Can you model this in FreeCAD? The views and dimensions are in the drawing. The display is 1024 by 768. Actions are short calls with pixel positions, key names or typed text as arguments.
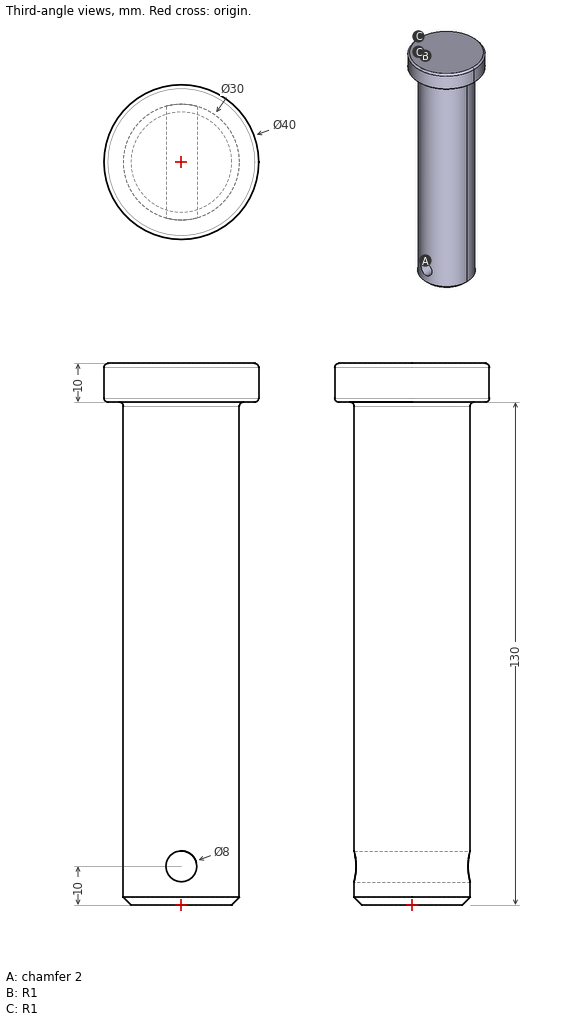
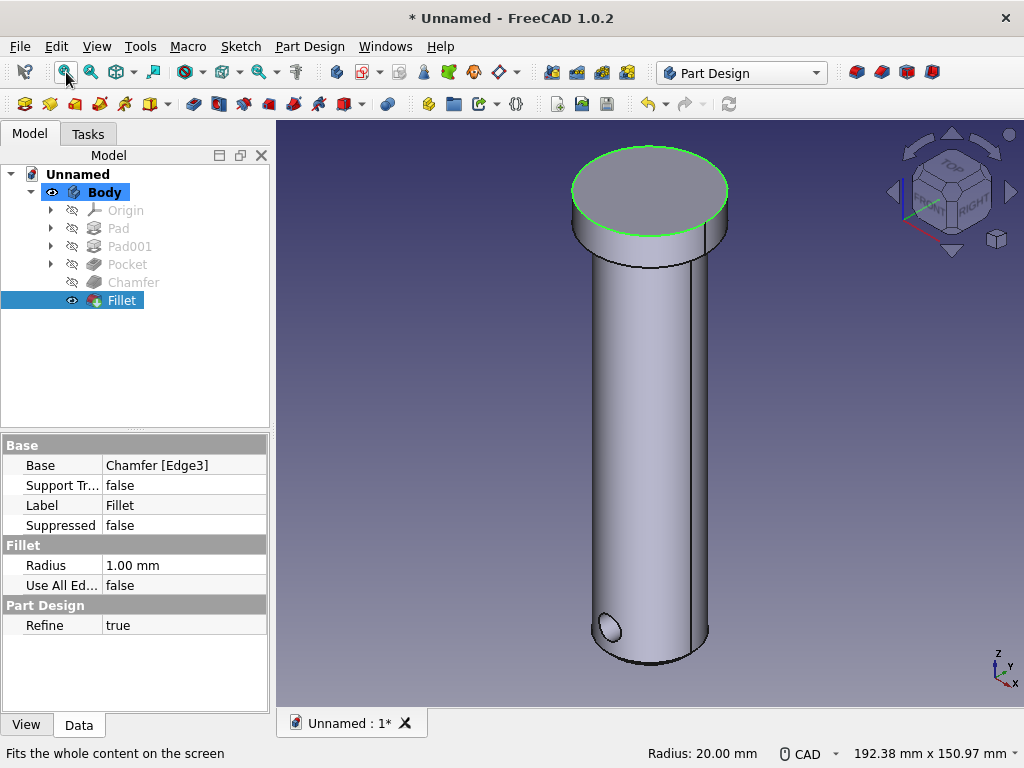
key(1)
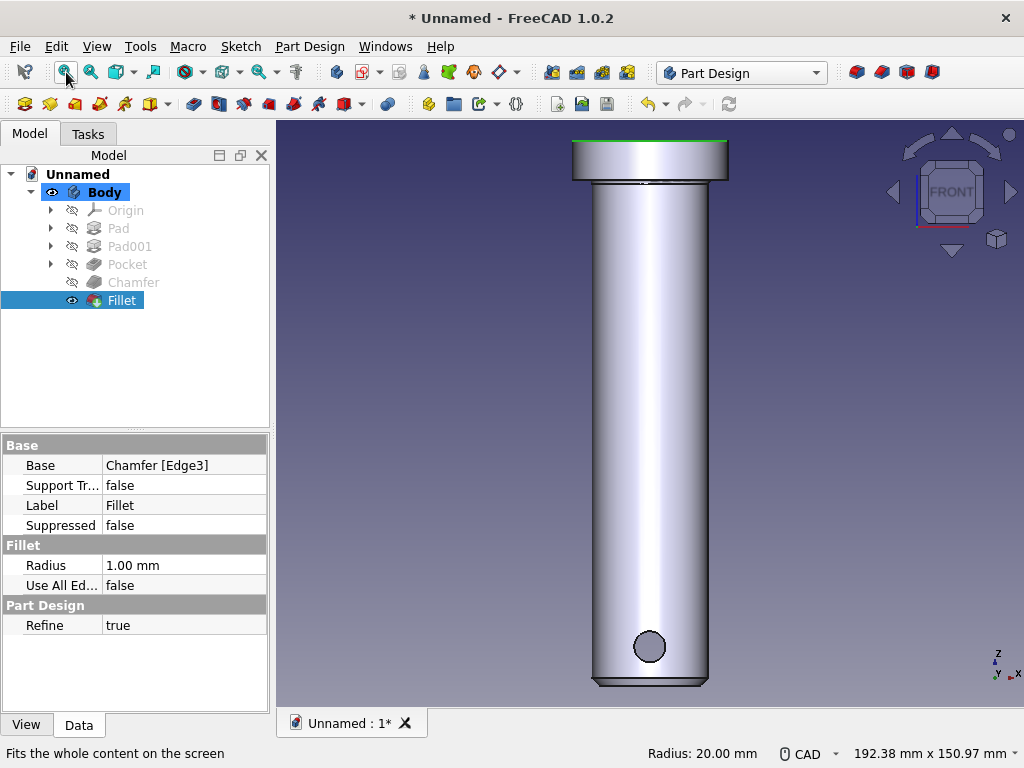
click(587, 179, ctrl)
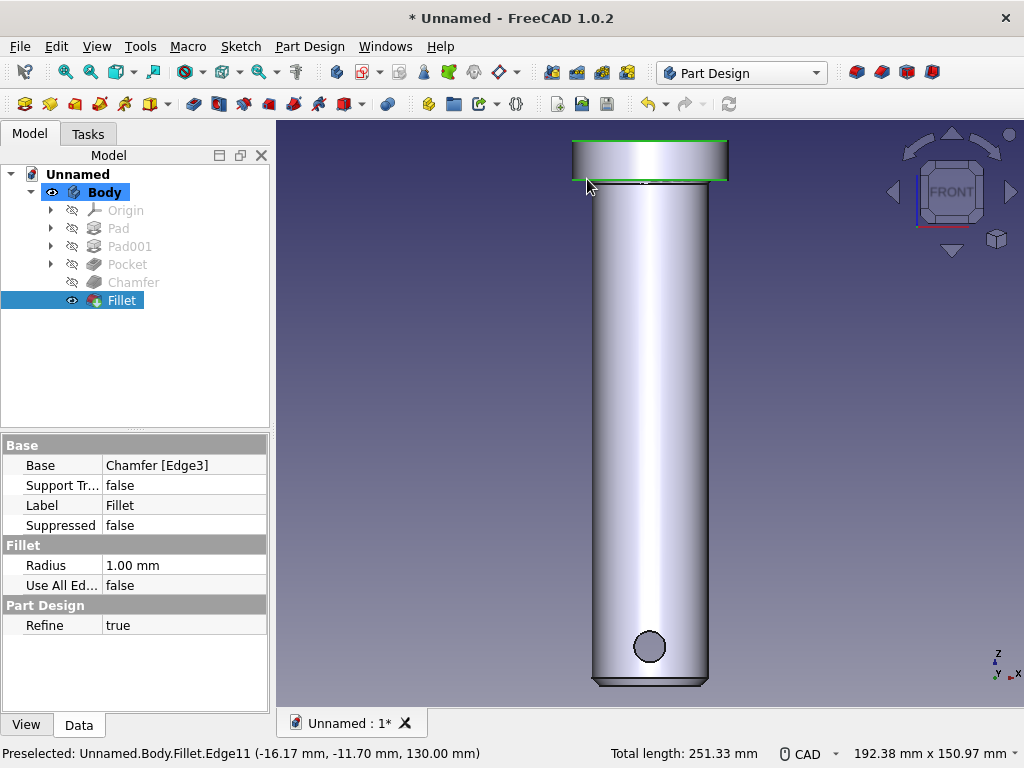
click(857, 72)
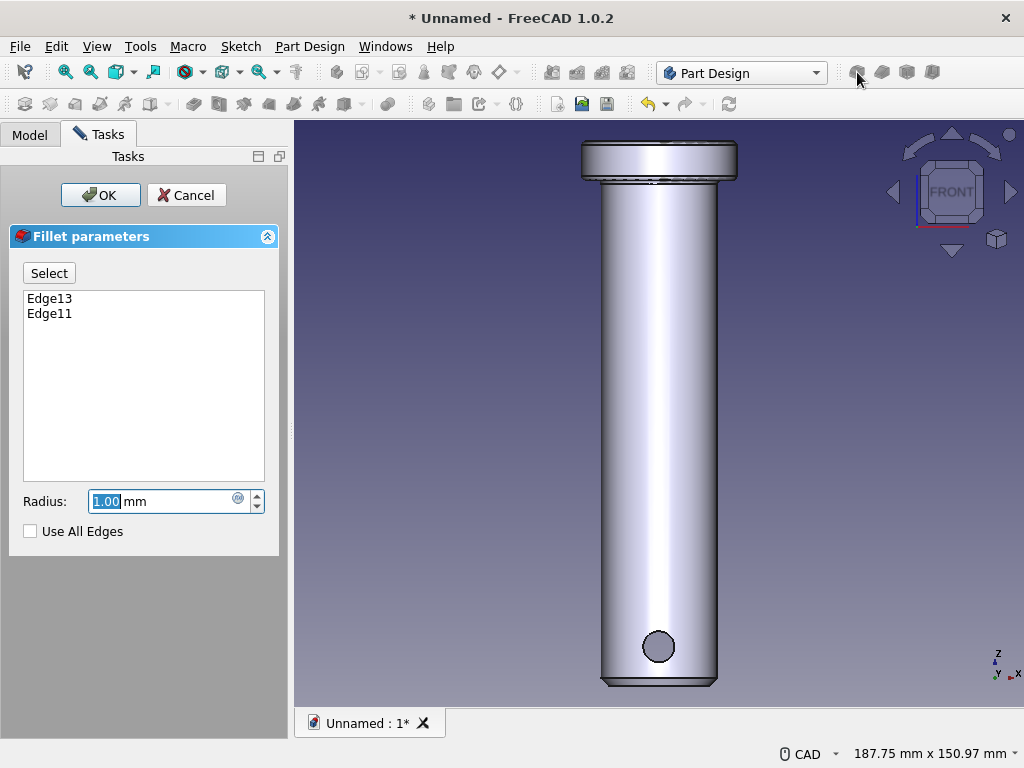
text(1)
key(Tab)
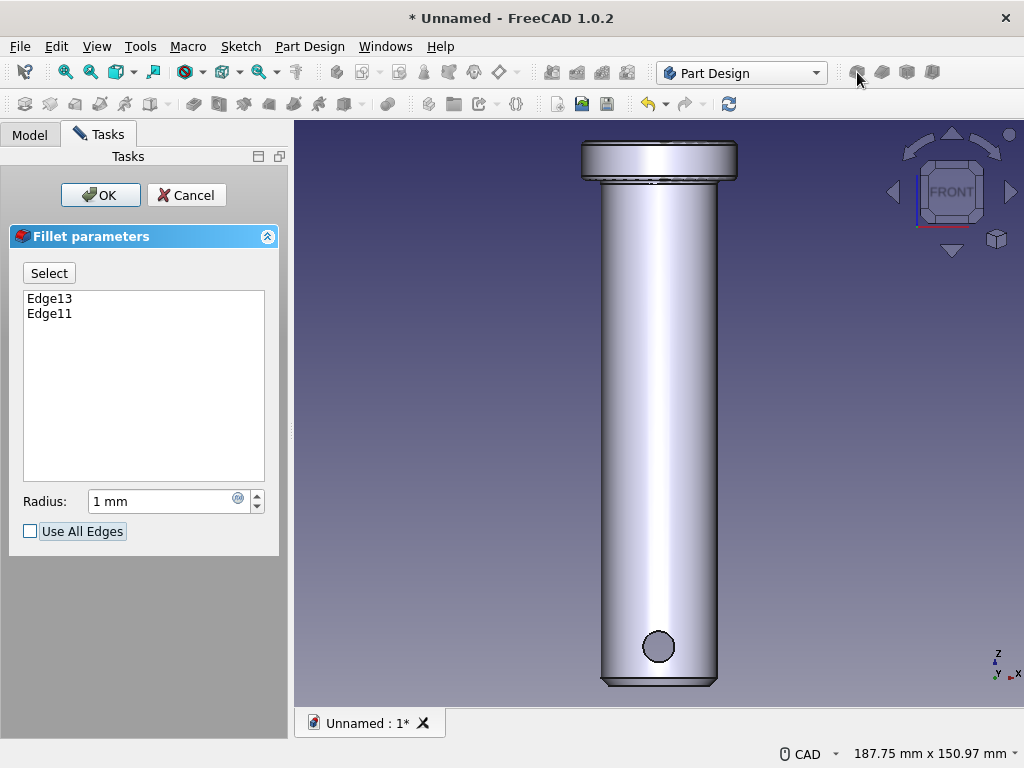
click(101, 195)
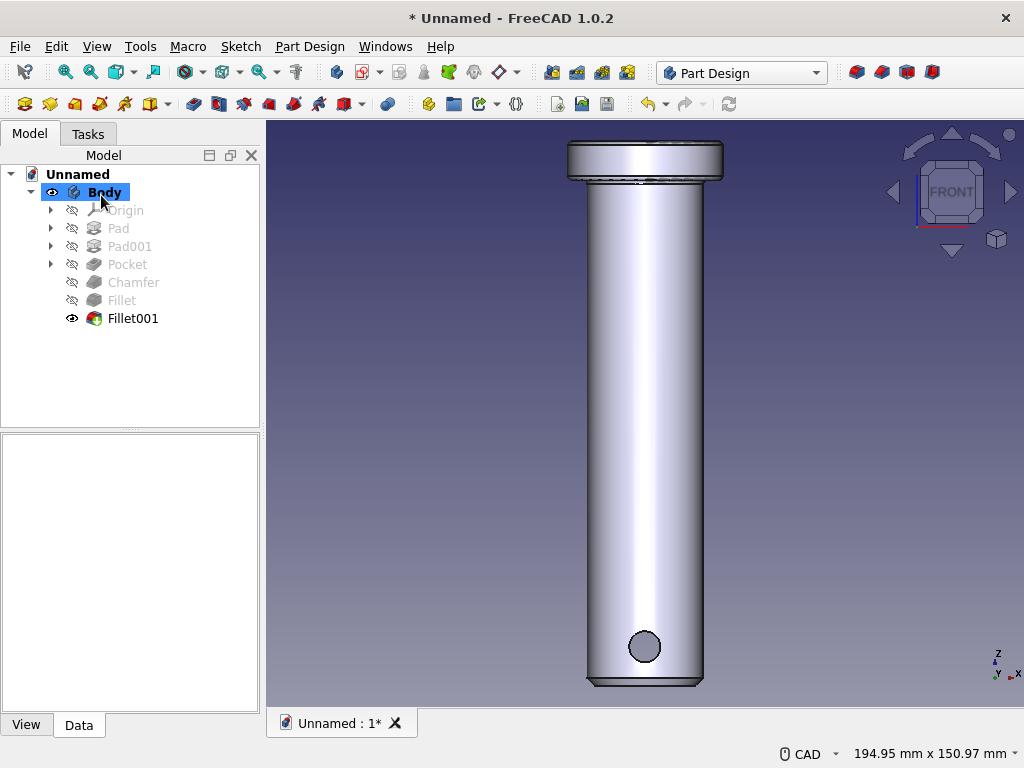
key(0)